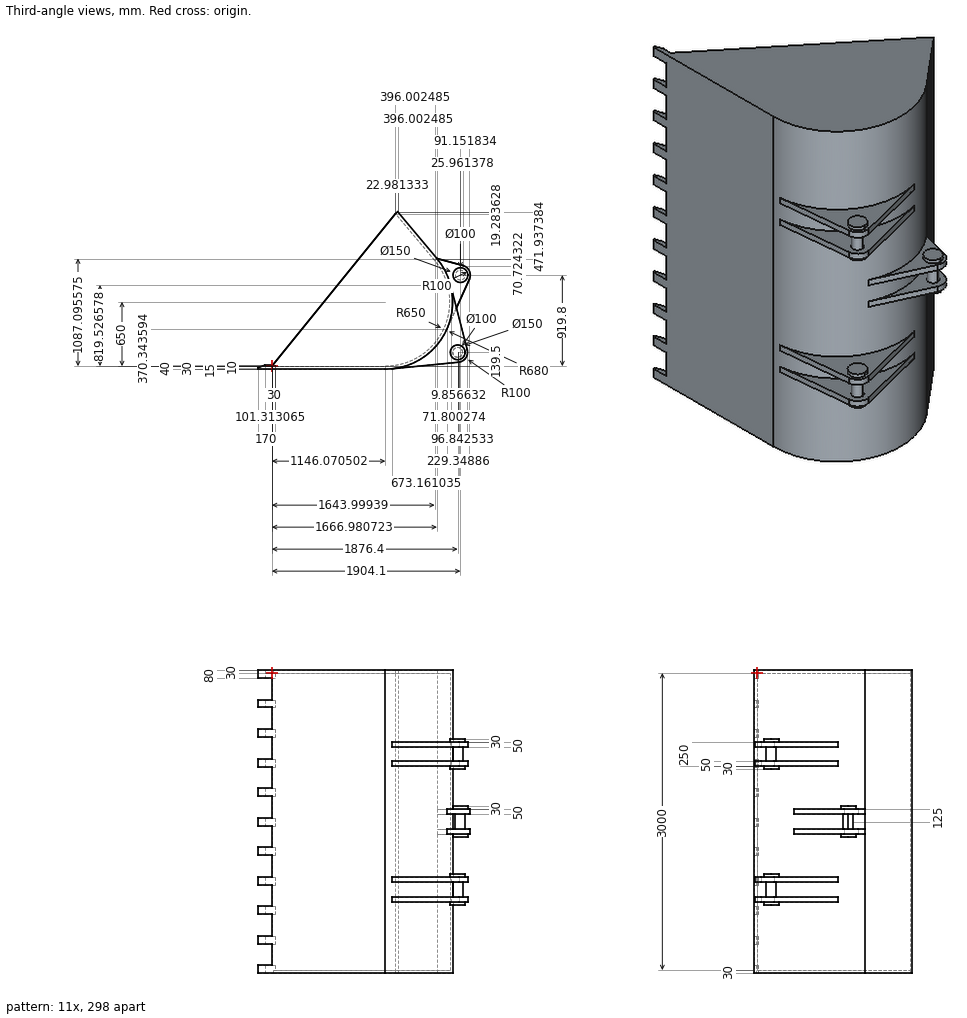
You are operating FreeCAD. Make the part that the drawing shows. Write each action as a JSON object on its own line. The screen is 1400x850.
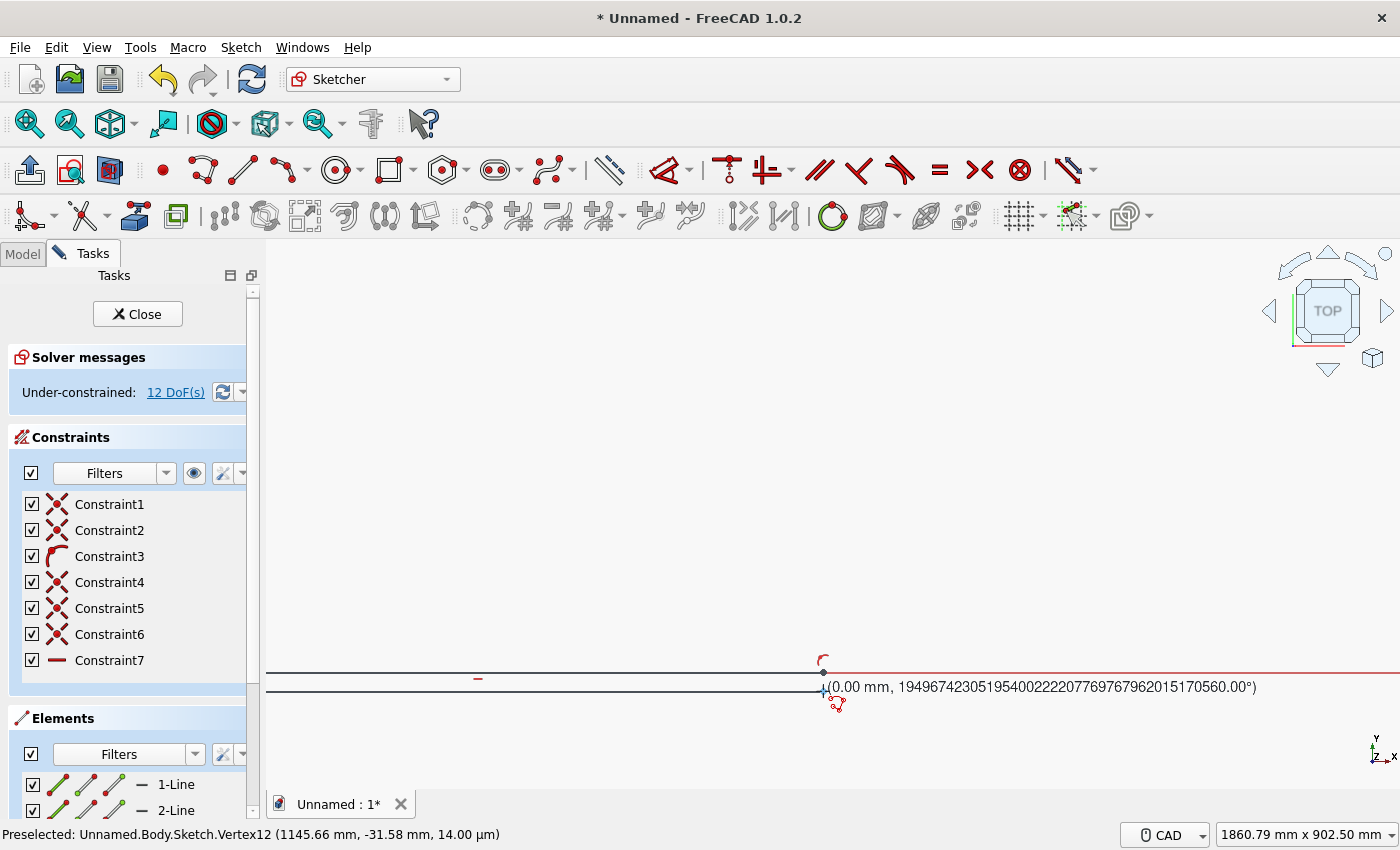
{"action": "left_click", "coordinate": [284, 170]}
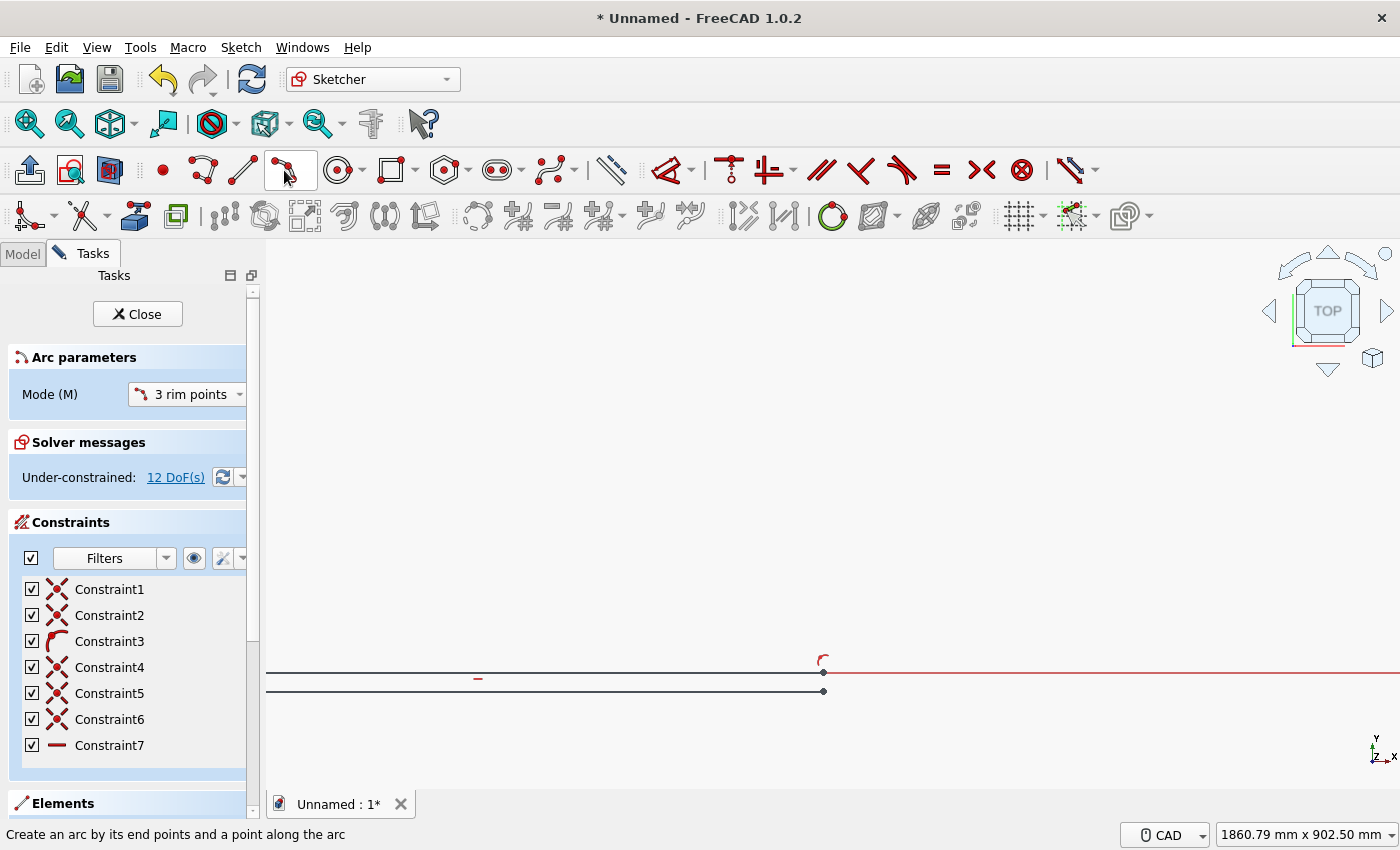
{"action": "scroll", "coordinate": [824, 693], "scroll_direction": "down", "scroll_amount": 5}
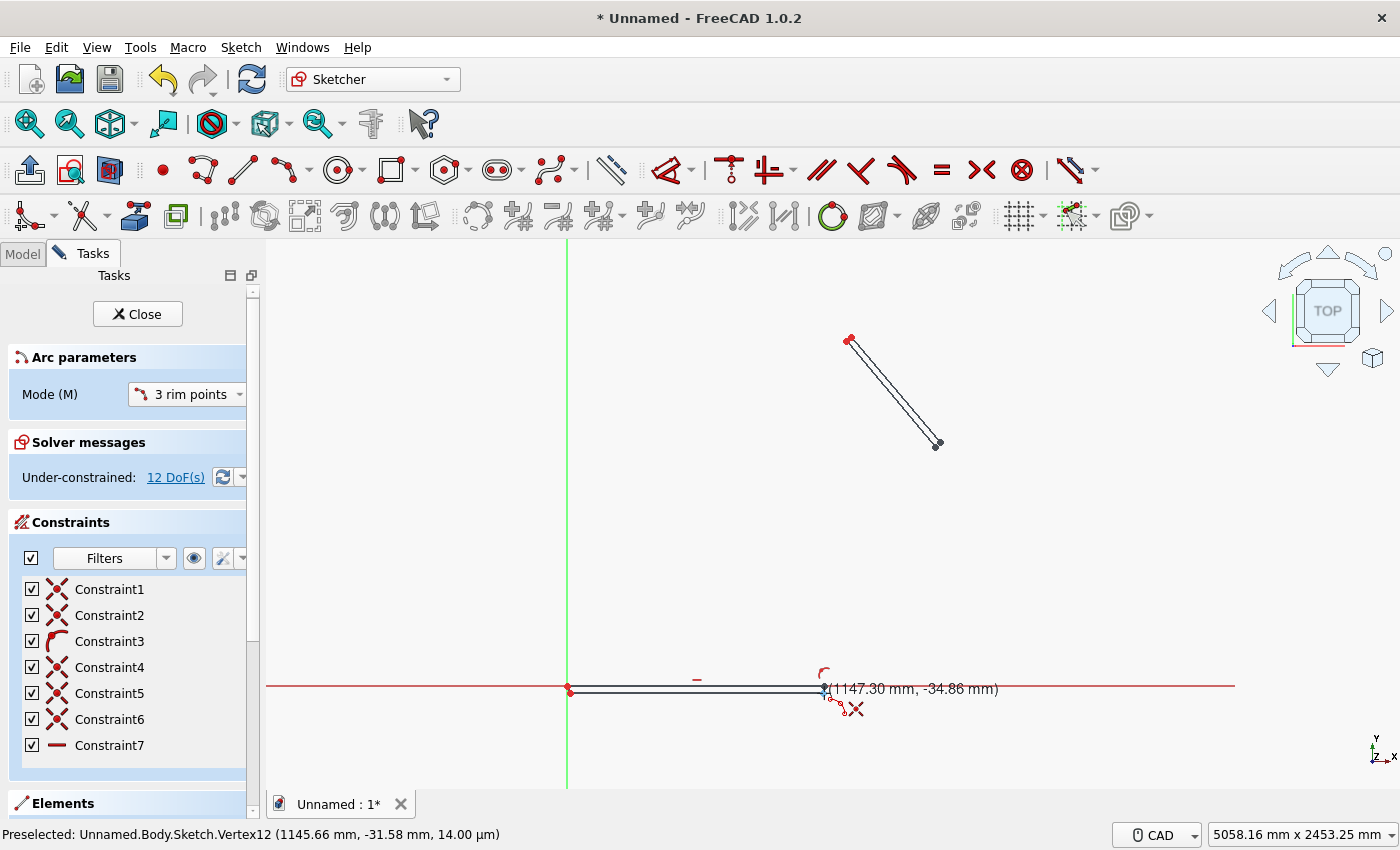
{"action": "scroll", "coordinate": [936, 447], "scroll_direction": "up", "scroll_amount": 5}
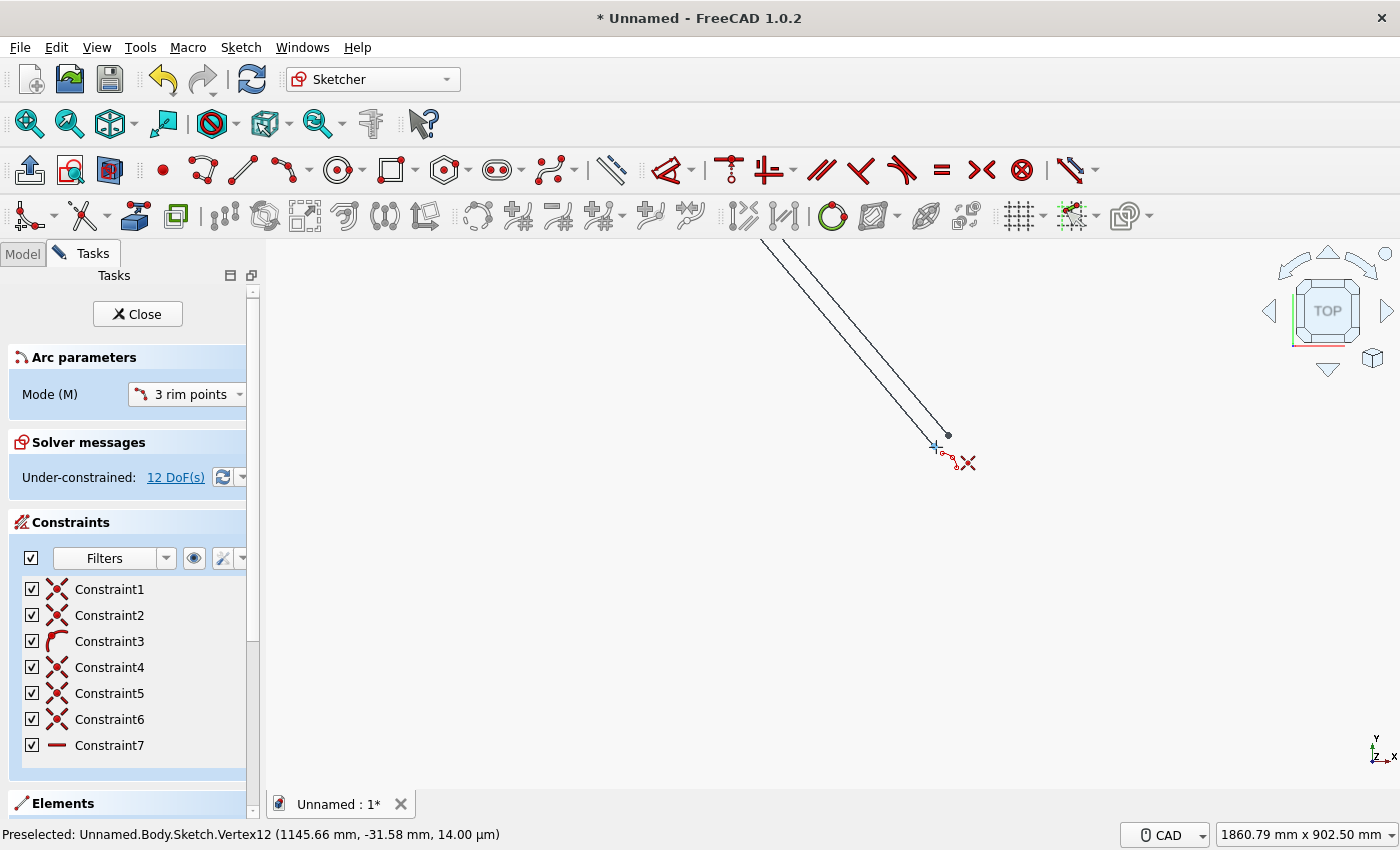
{"action": "left_click", "coordinate": [934, 446]}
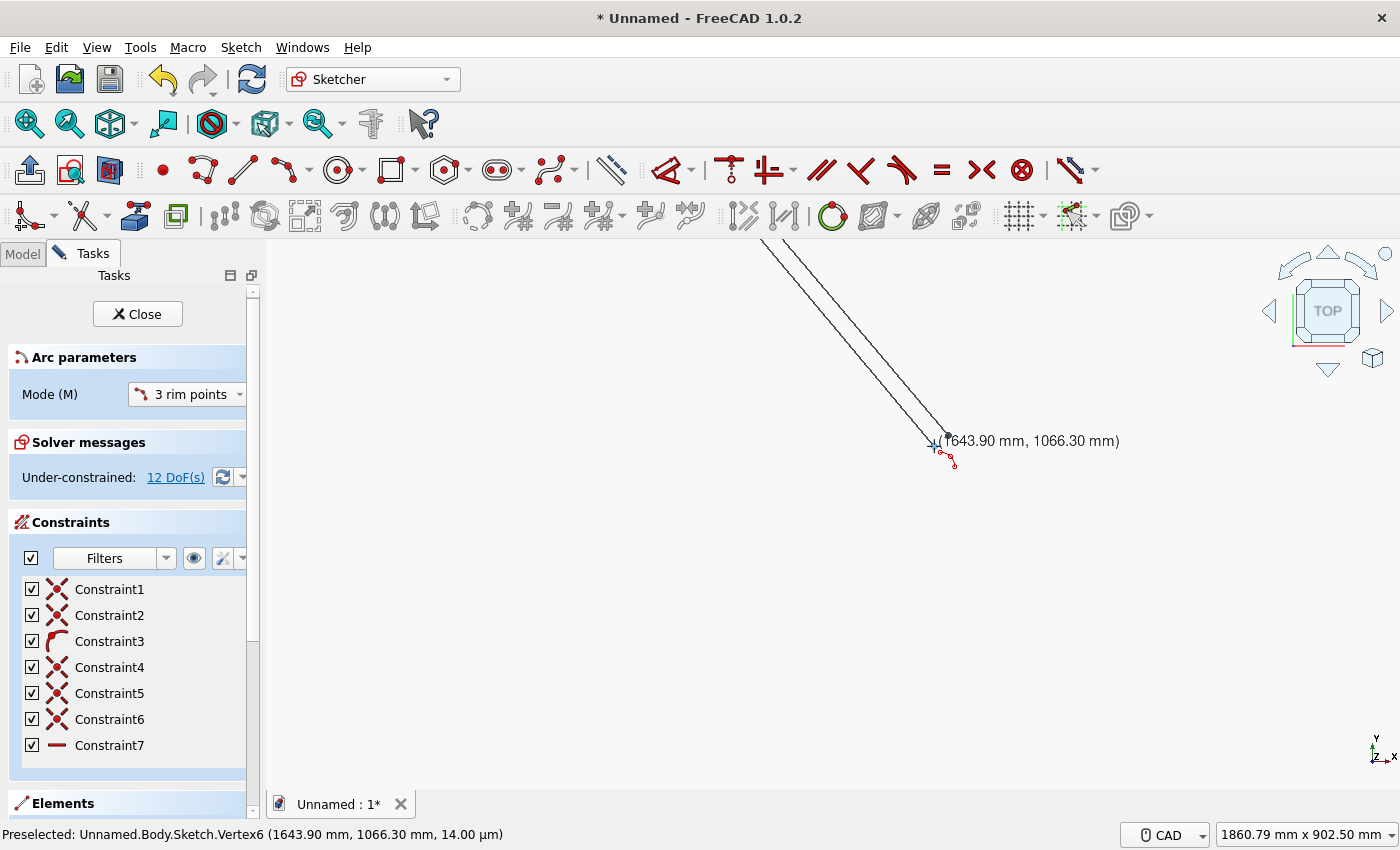
{"action": "scroll", "coordinate": [936, 446], "scroll_direction": "down", "scroll_amount": 5}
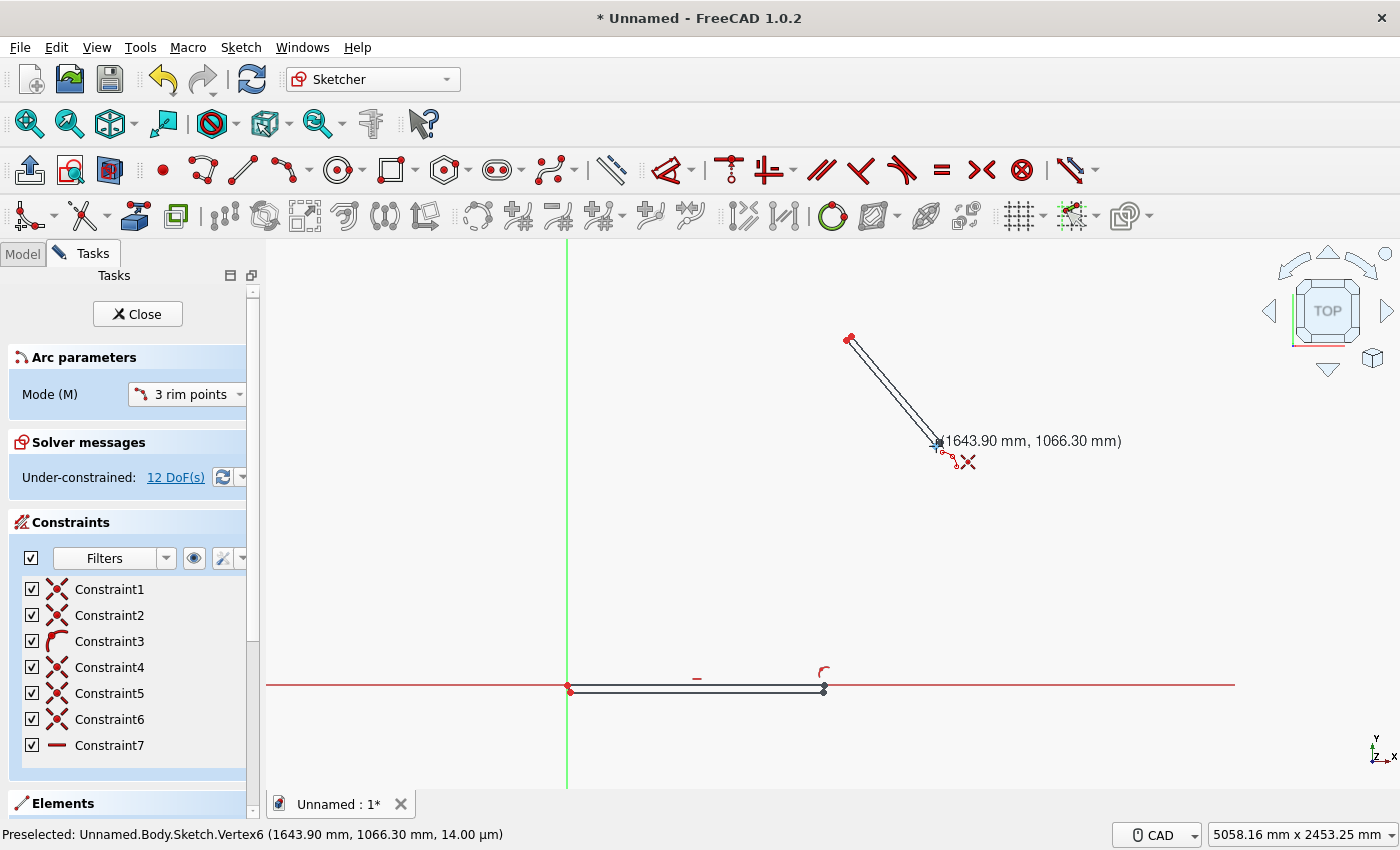
{"action": "scroll", "coordinate": [824, 685], "scroll_direction": "up", "scroll_amount": 5}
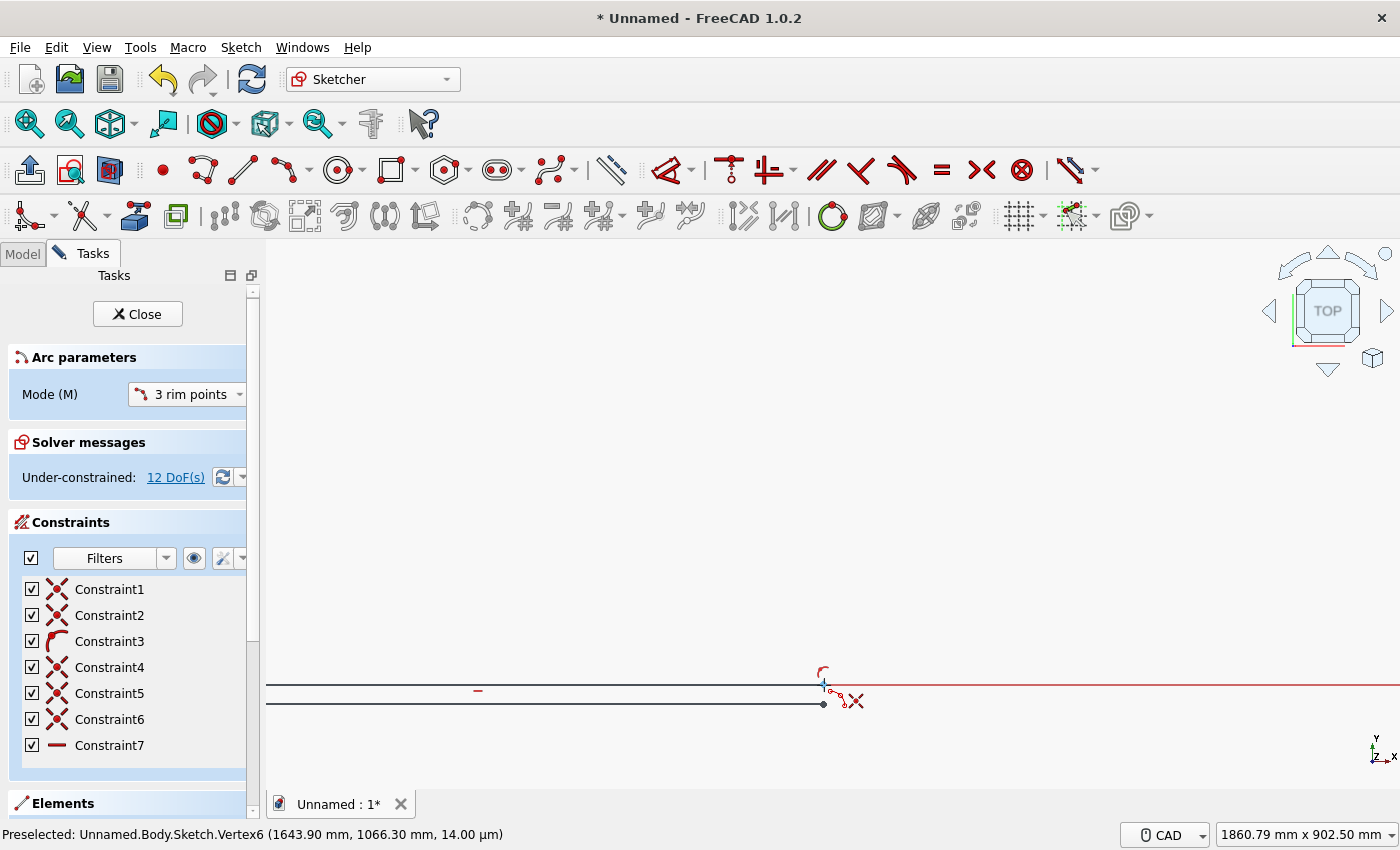
{"action": "left_click", "coordinate": [823, 685]}
{"action": "left_click", "coordinate": [1182, 456]}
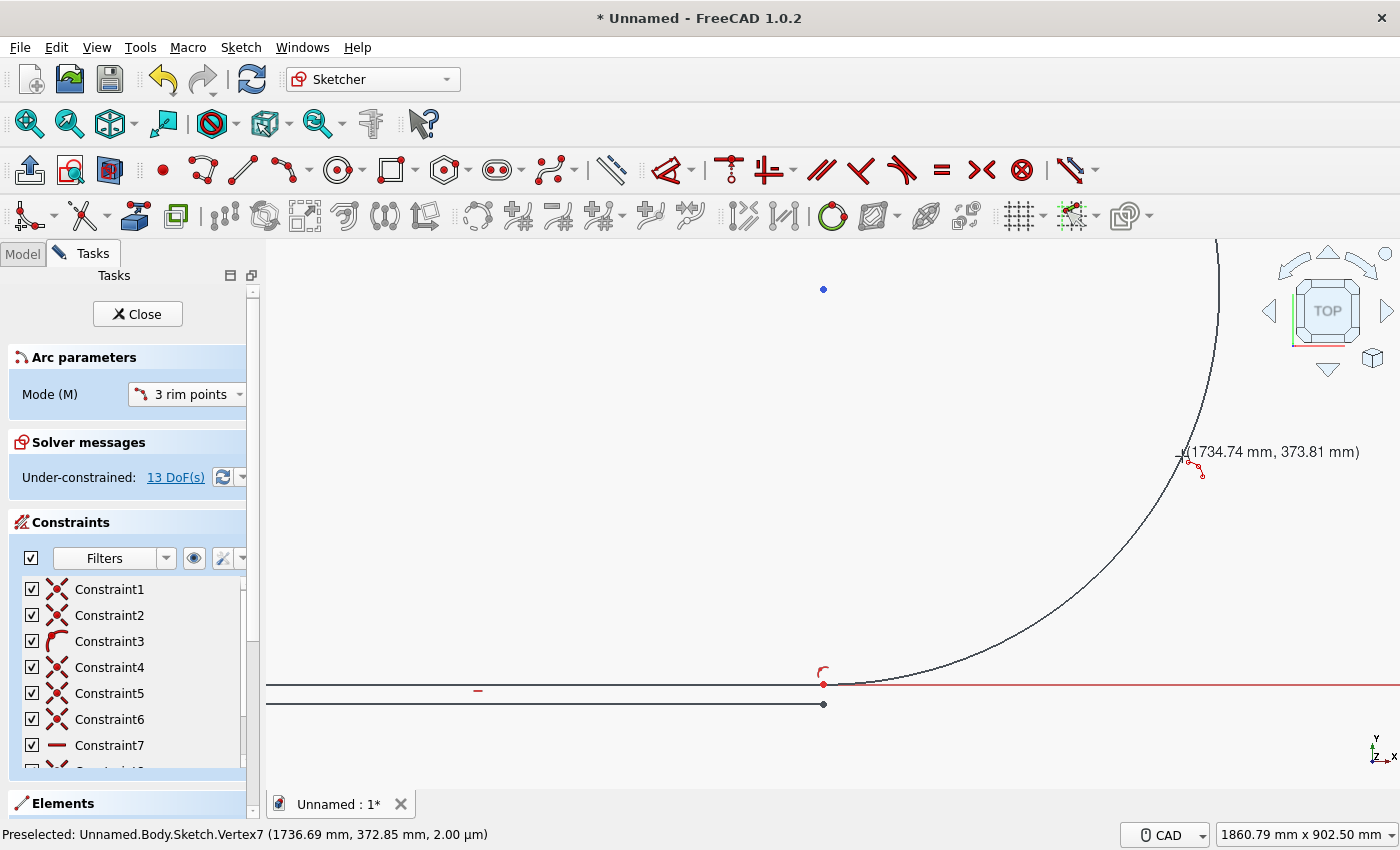
{"action": "left_click", "coordinate": [823, 704]}